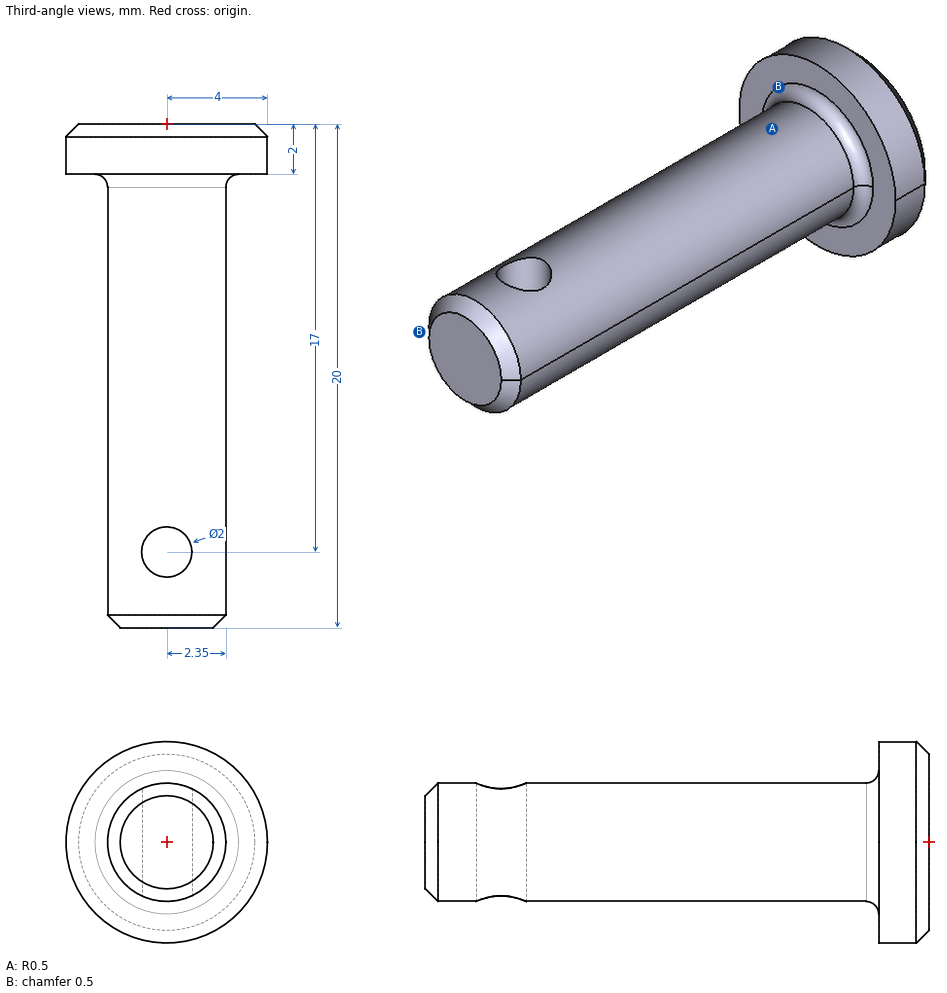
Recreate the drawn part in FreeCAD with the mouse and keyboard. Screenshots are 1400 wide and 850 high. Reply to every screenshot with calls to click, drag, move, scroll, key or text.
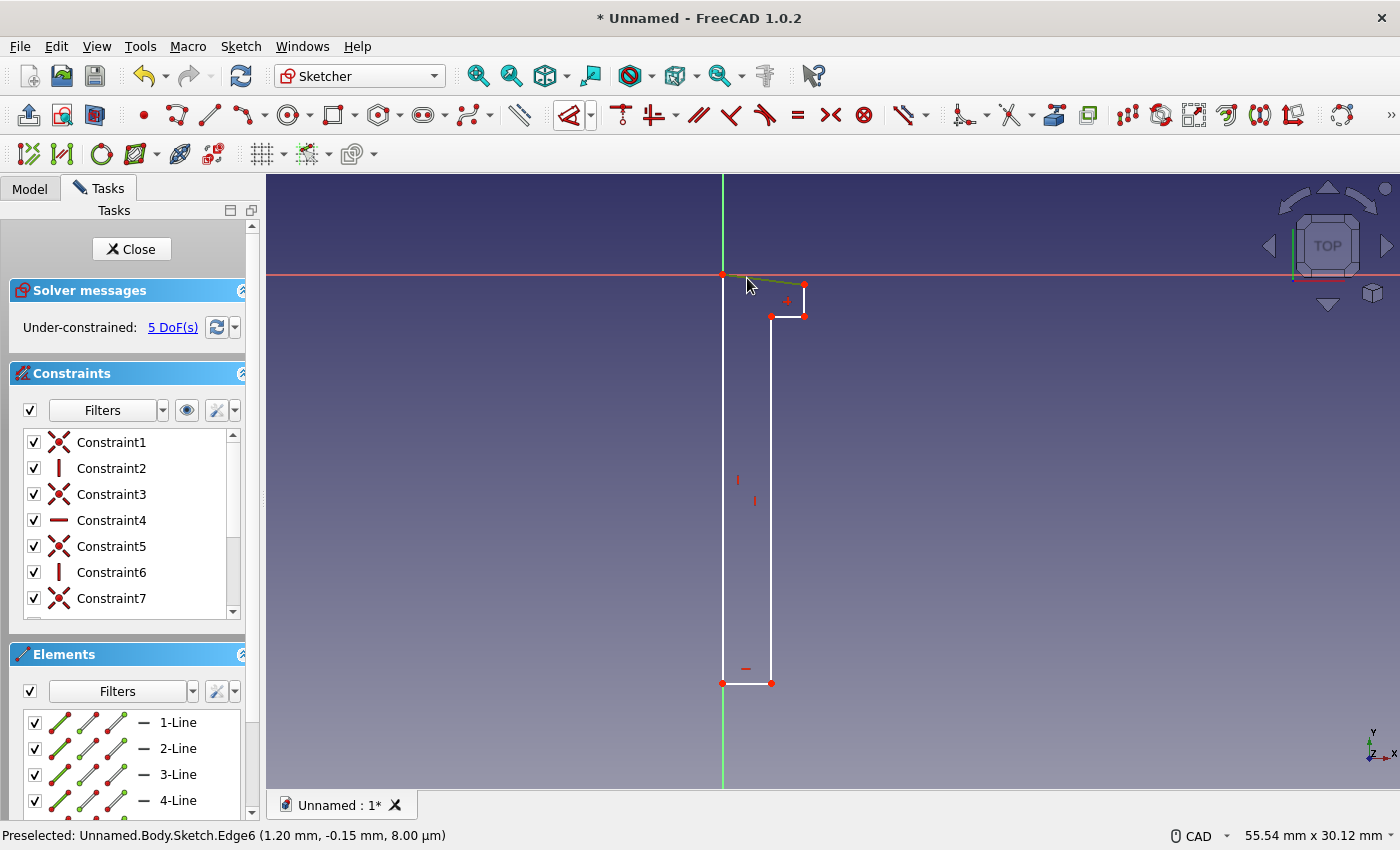
click(676, 116)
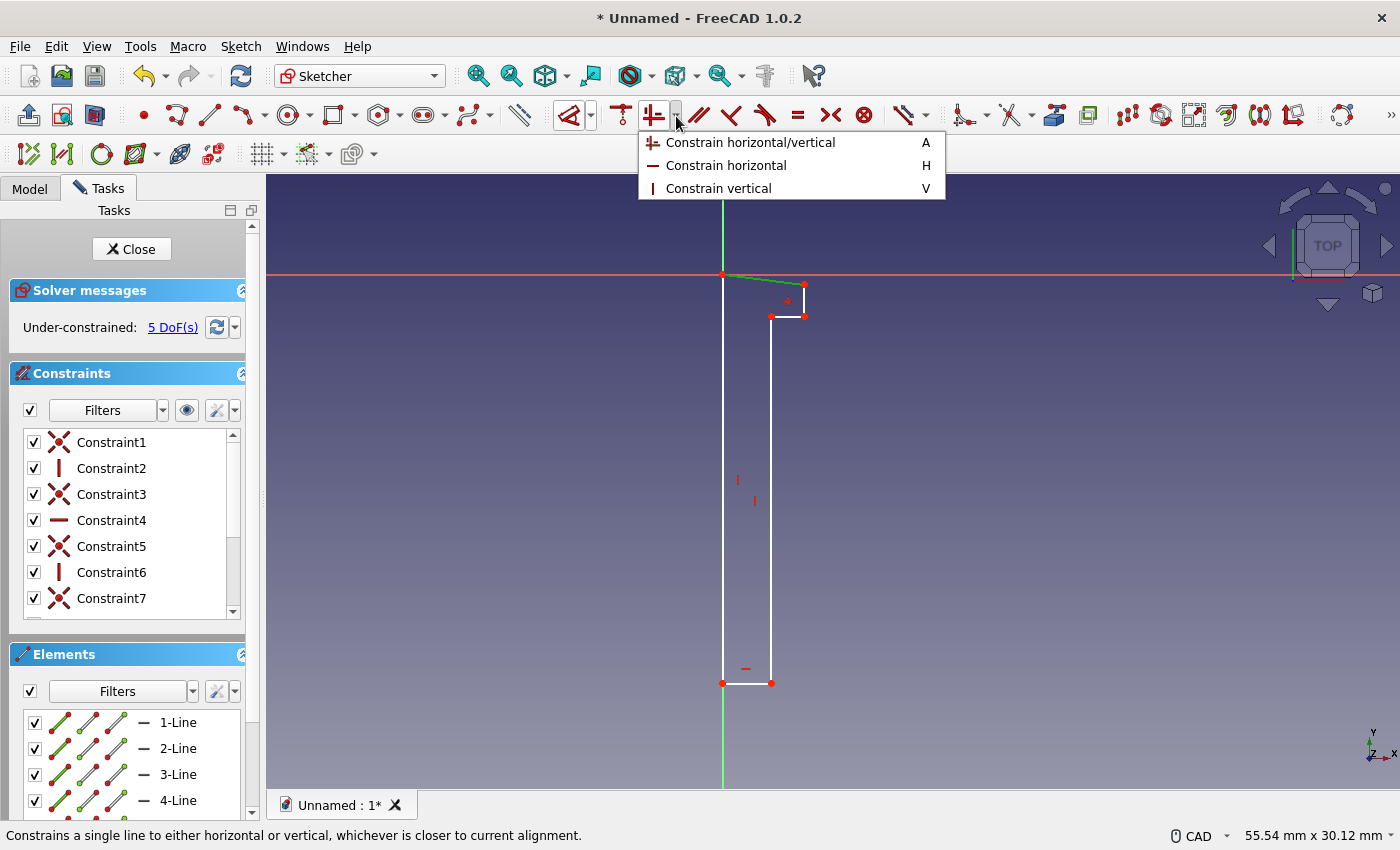
click(792, 166)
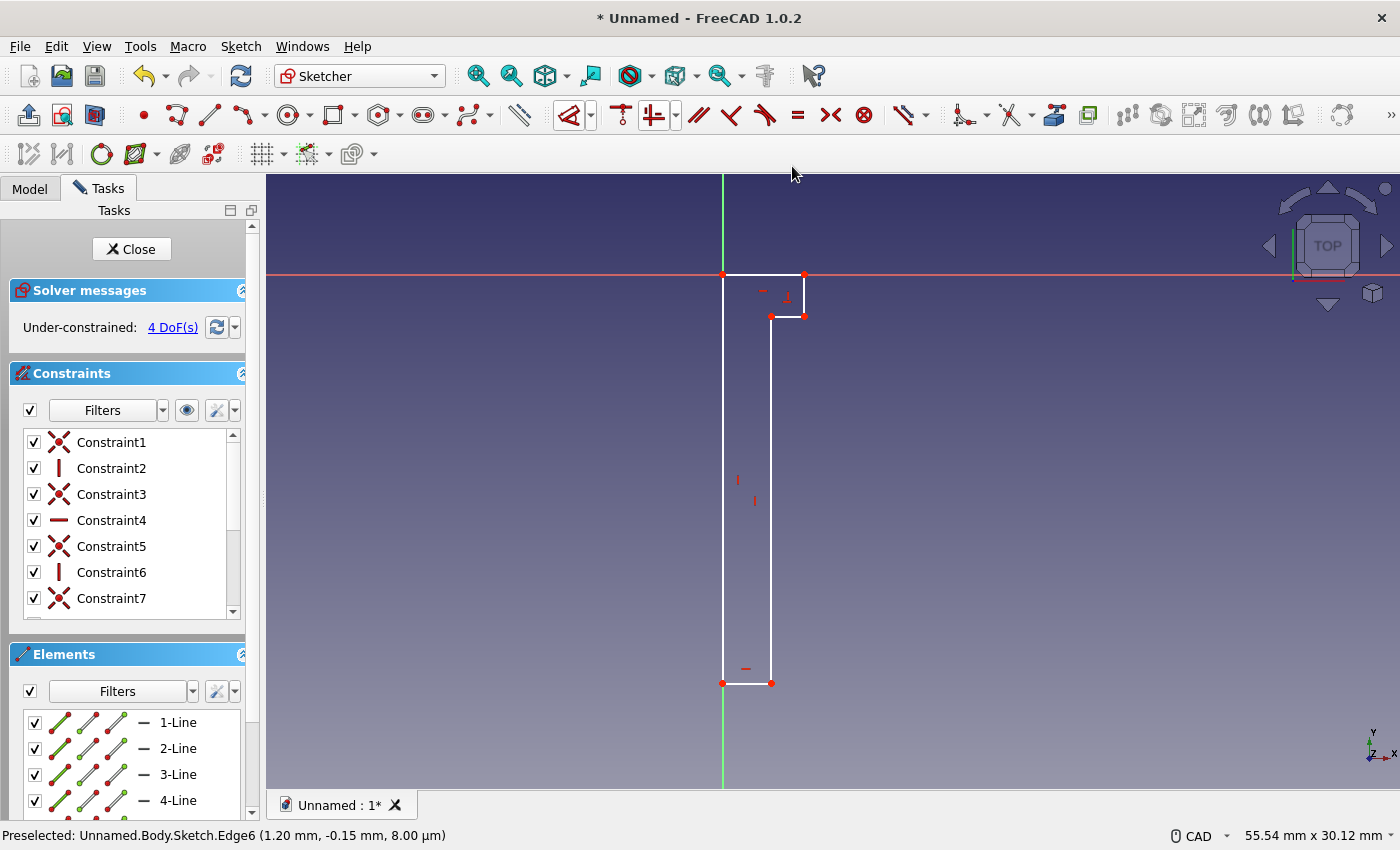
key(d)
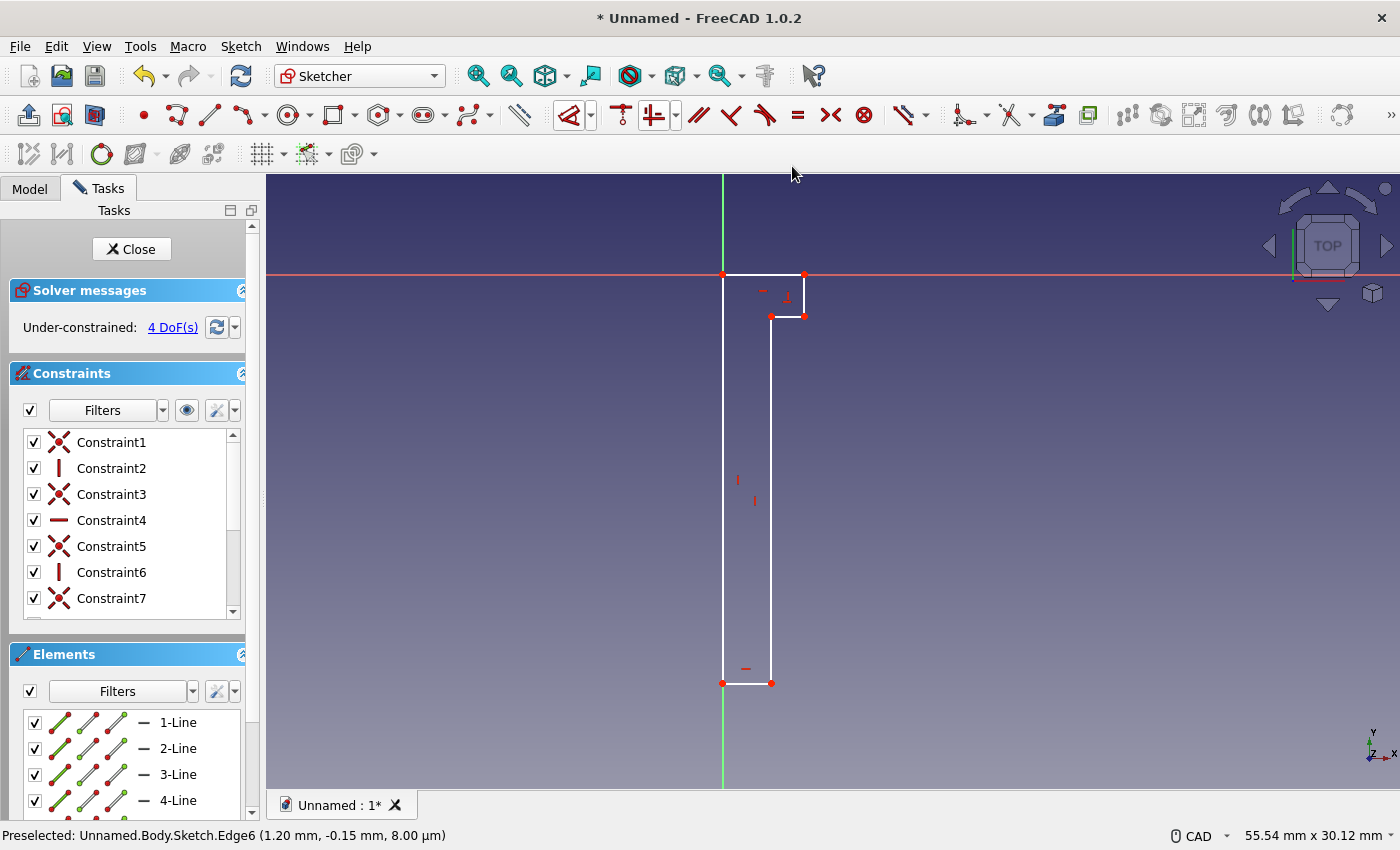
click(804, 304)
click(838, 296)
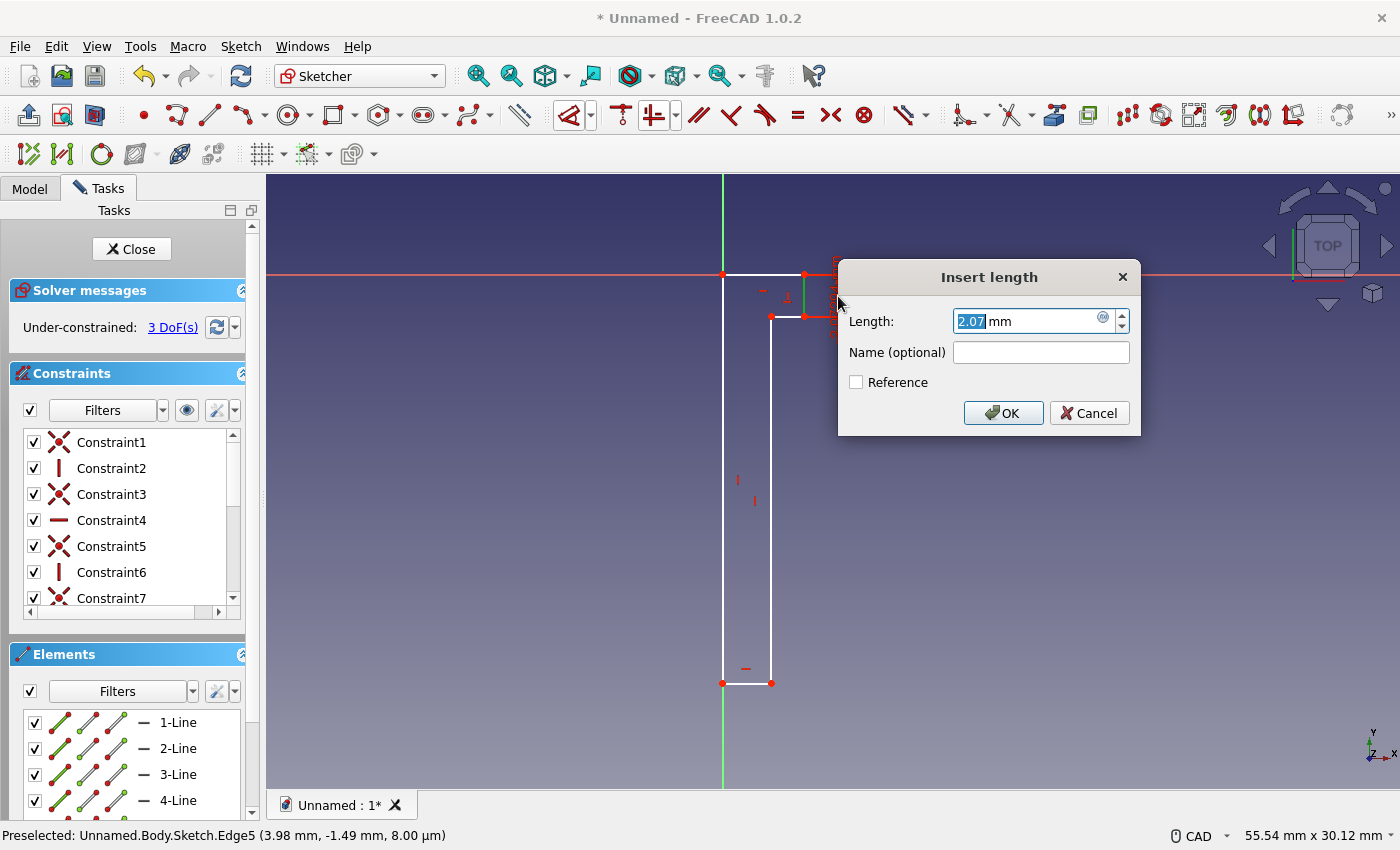
text(2)
key(Return)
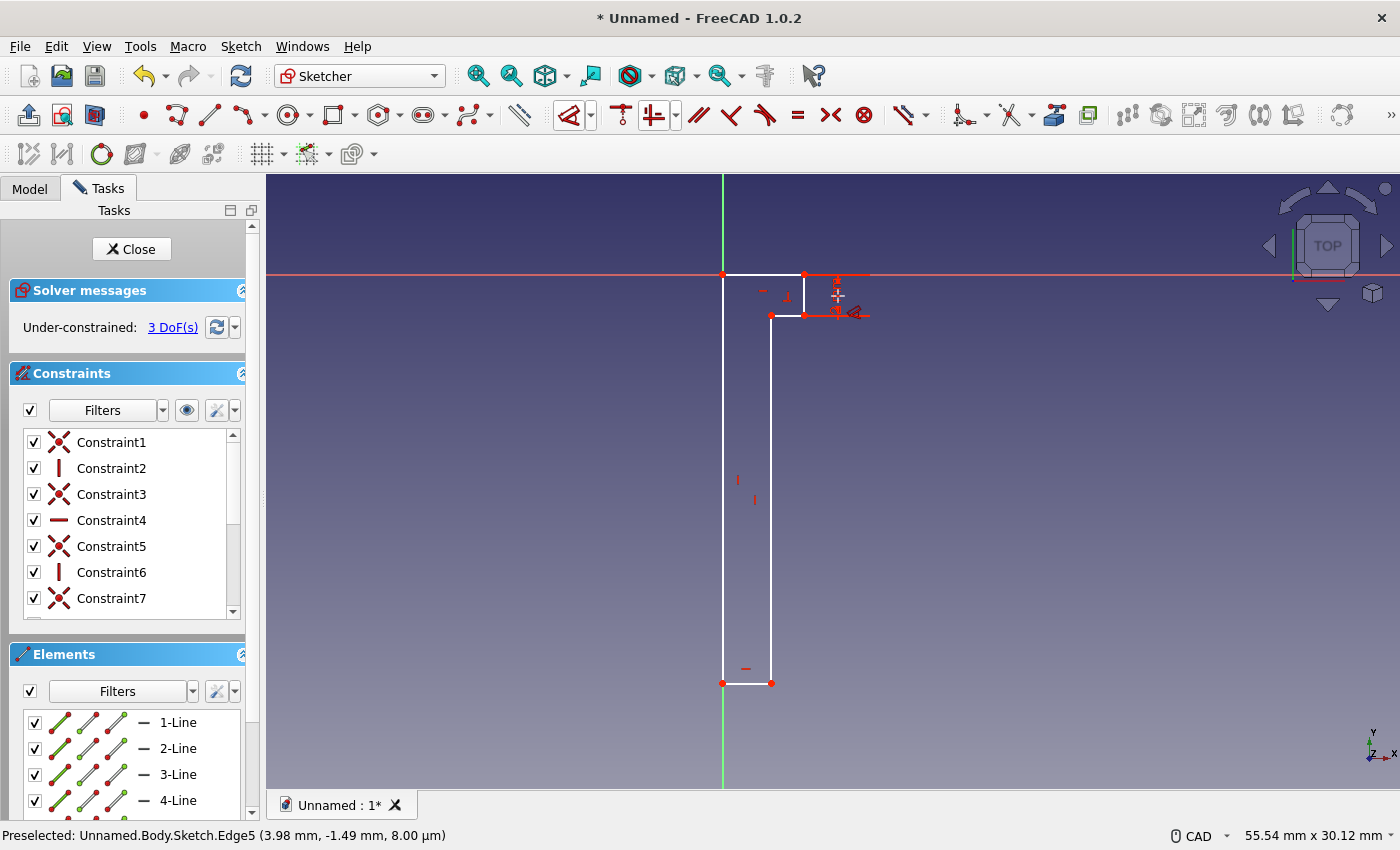
click(780, 275)
click(763, 241)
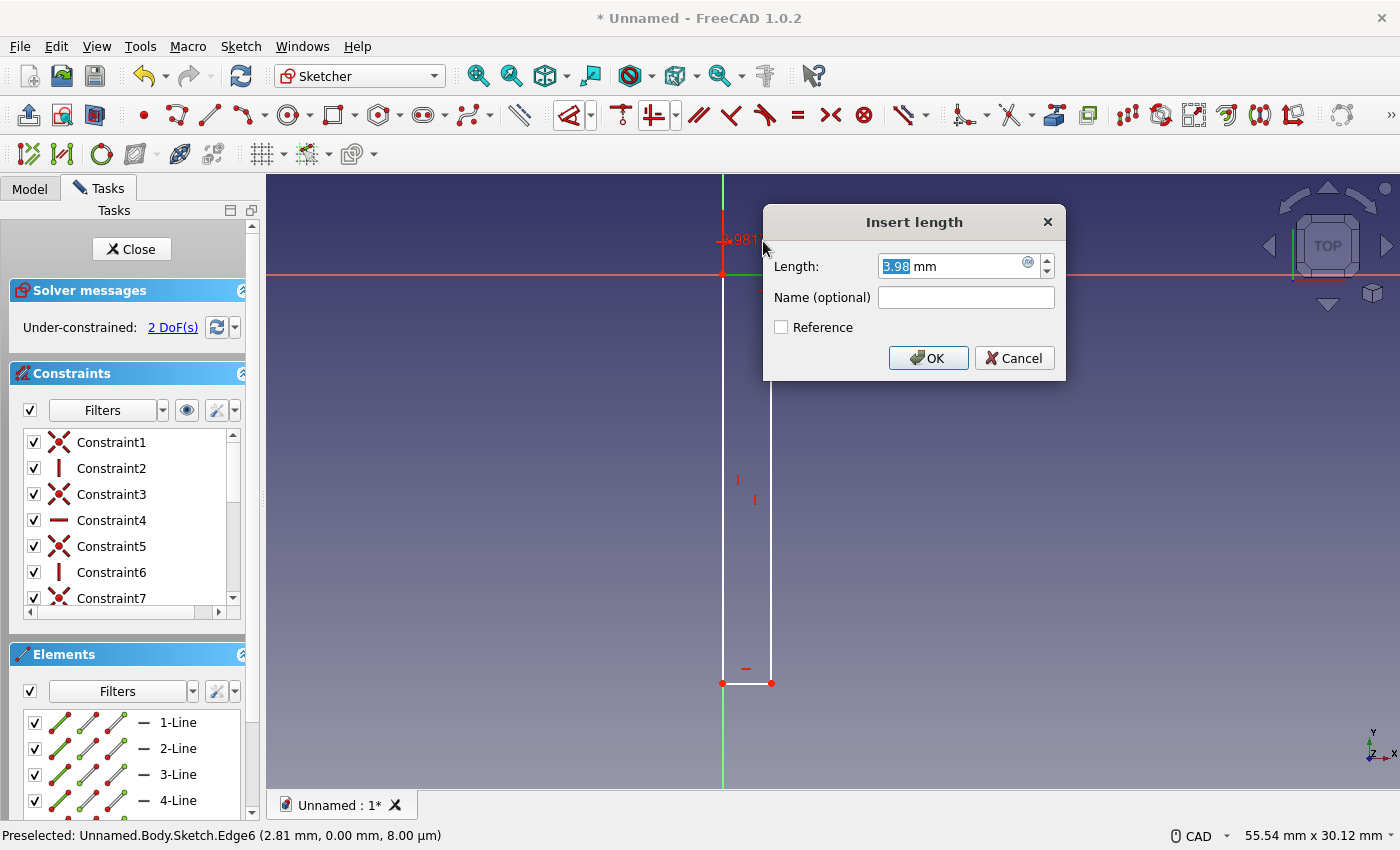
text(4)
key(Return)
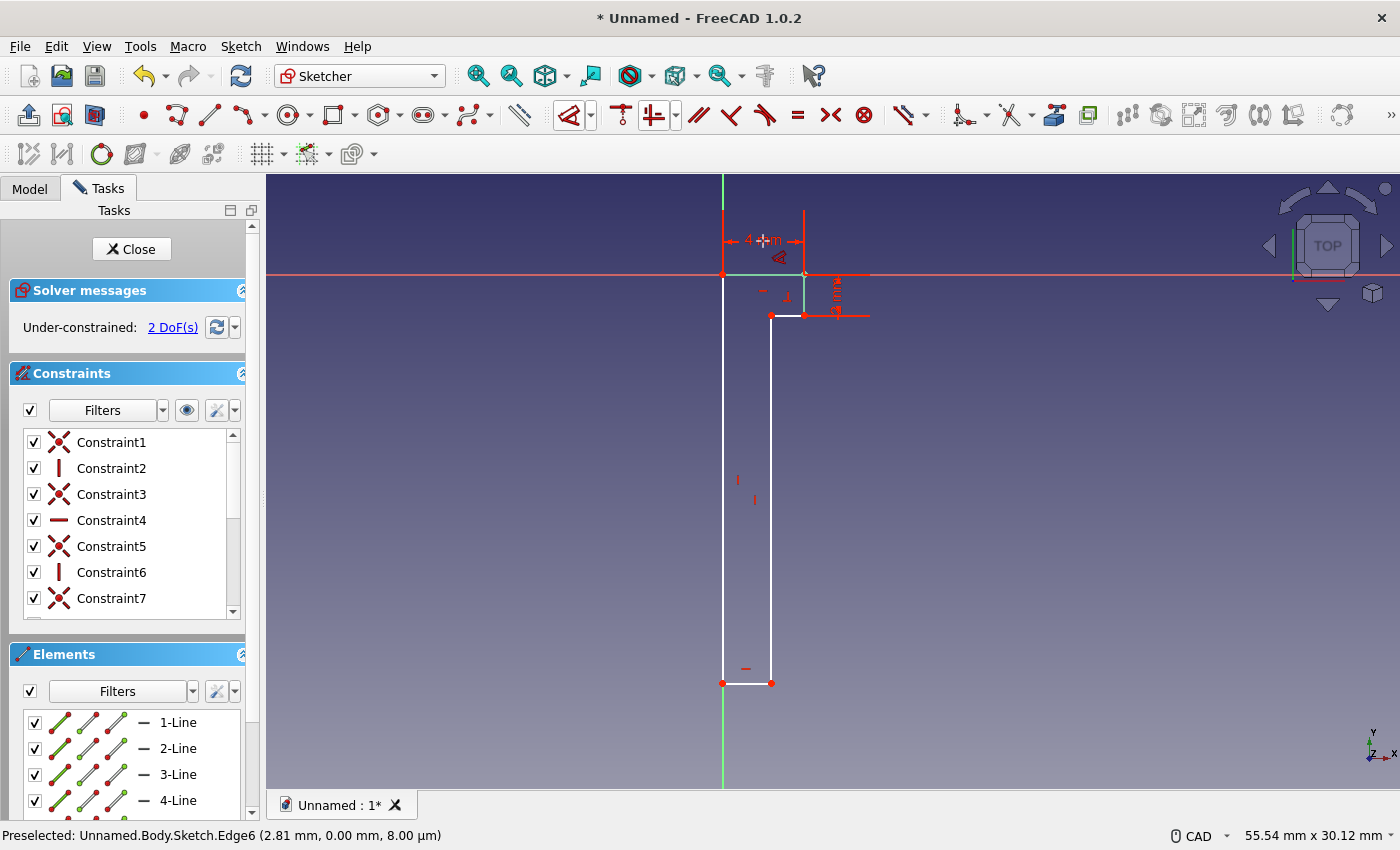
click(723, 397)
click(689, 479)